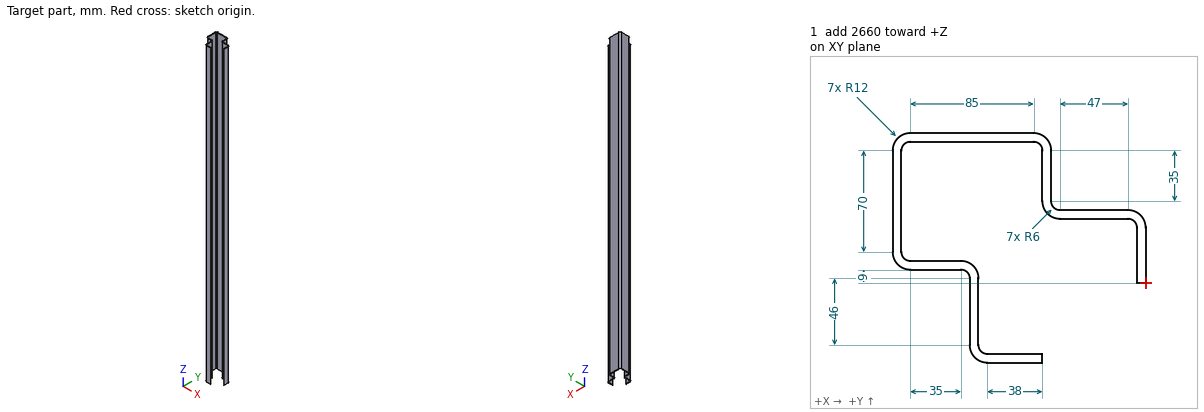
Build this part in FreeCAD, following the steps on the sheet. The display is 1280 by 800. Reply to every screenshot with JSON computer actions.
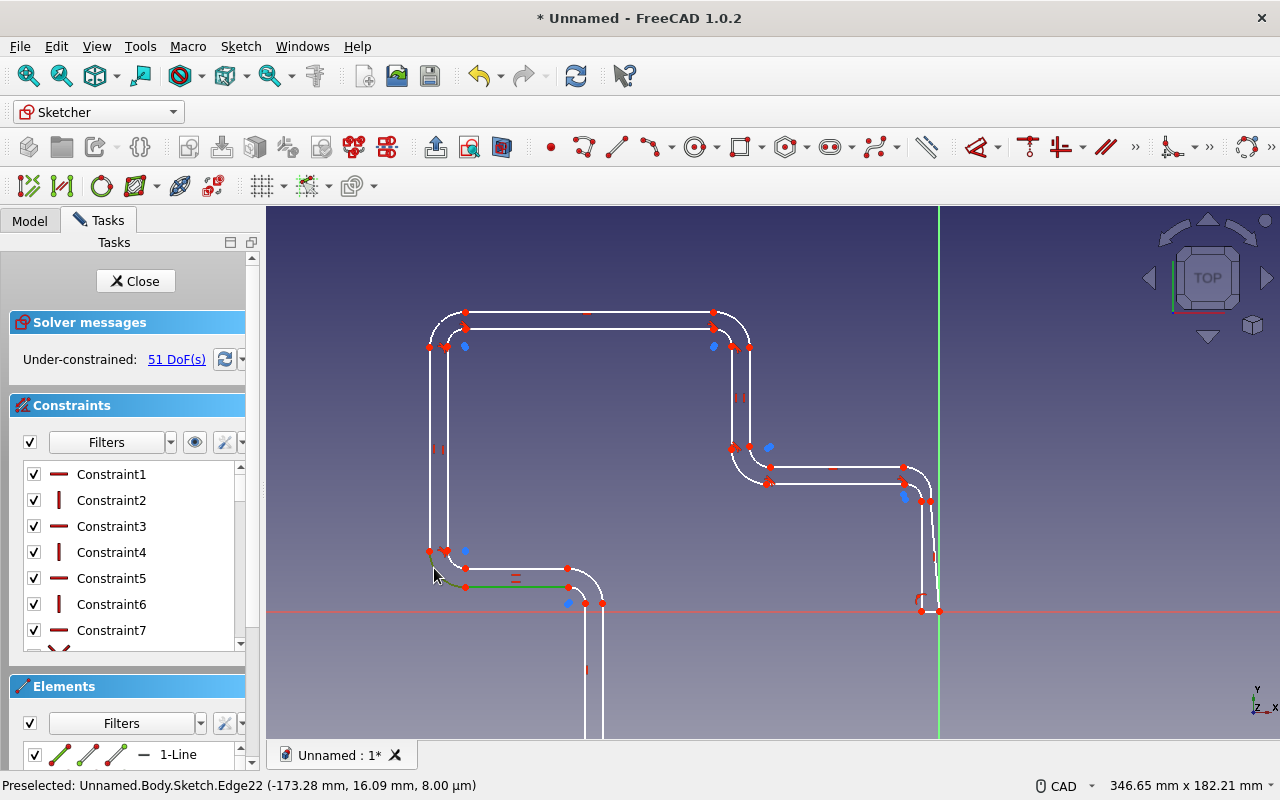
{"action": "key", "text": "t"}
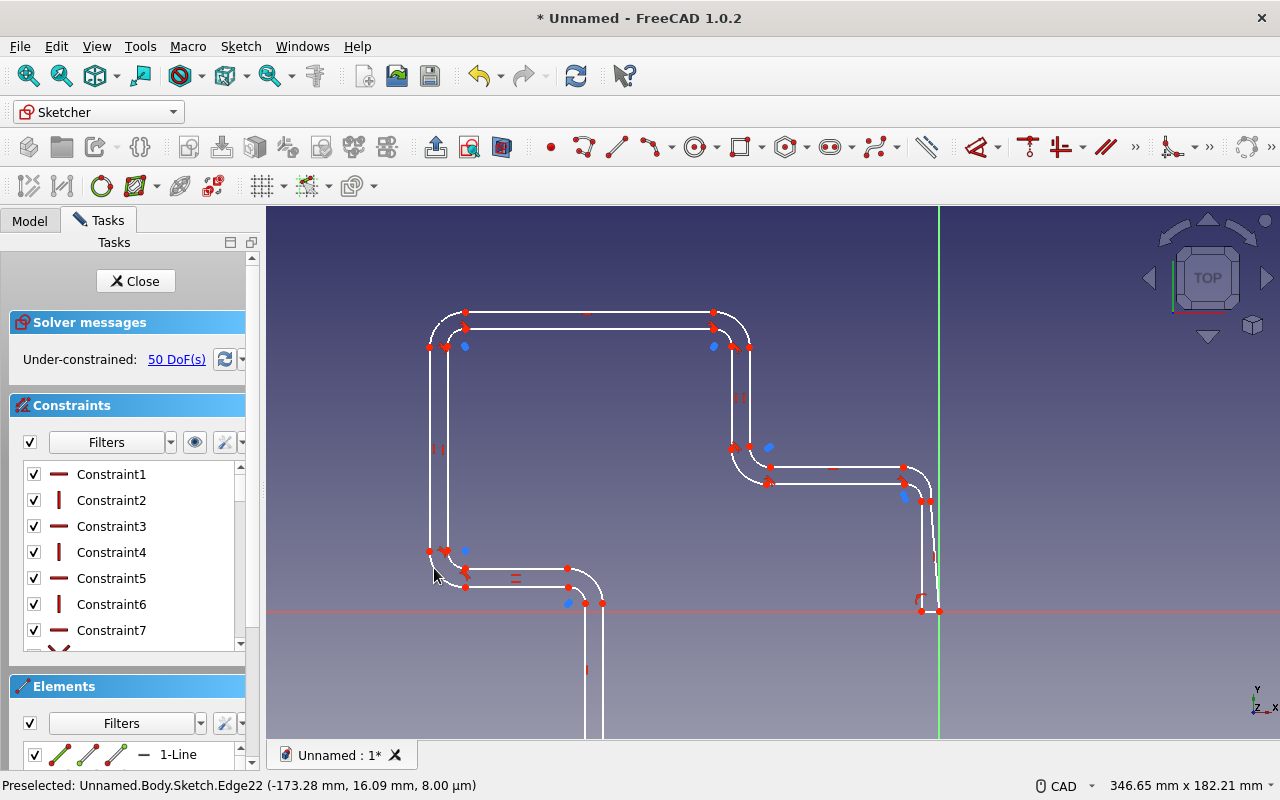
{"action": "left_click", "coordinate": [496, 587]}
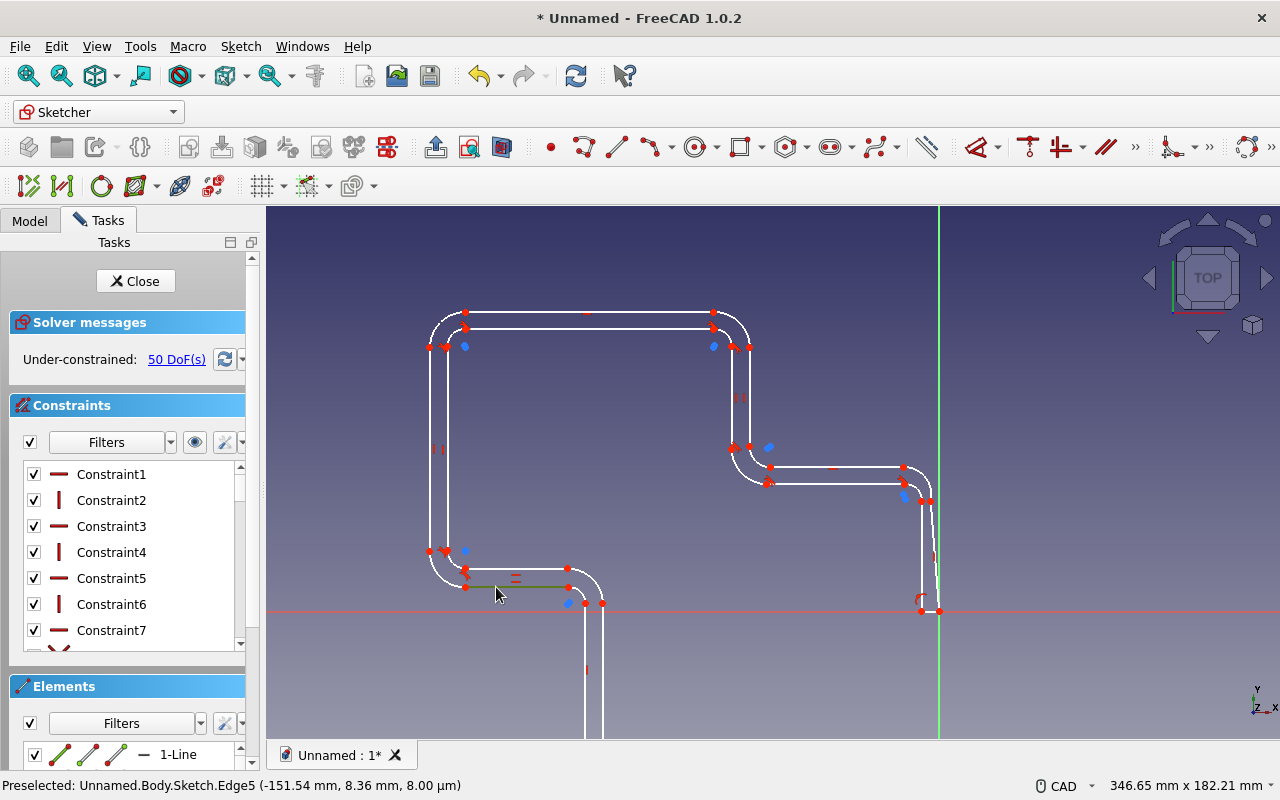
{"action": "left_click", "coordinate": [580, 592]}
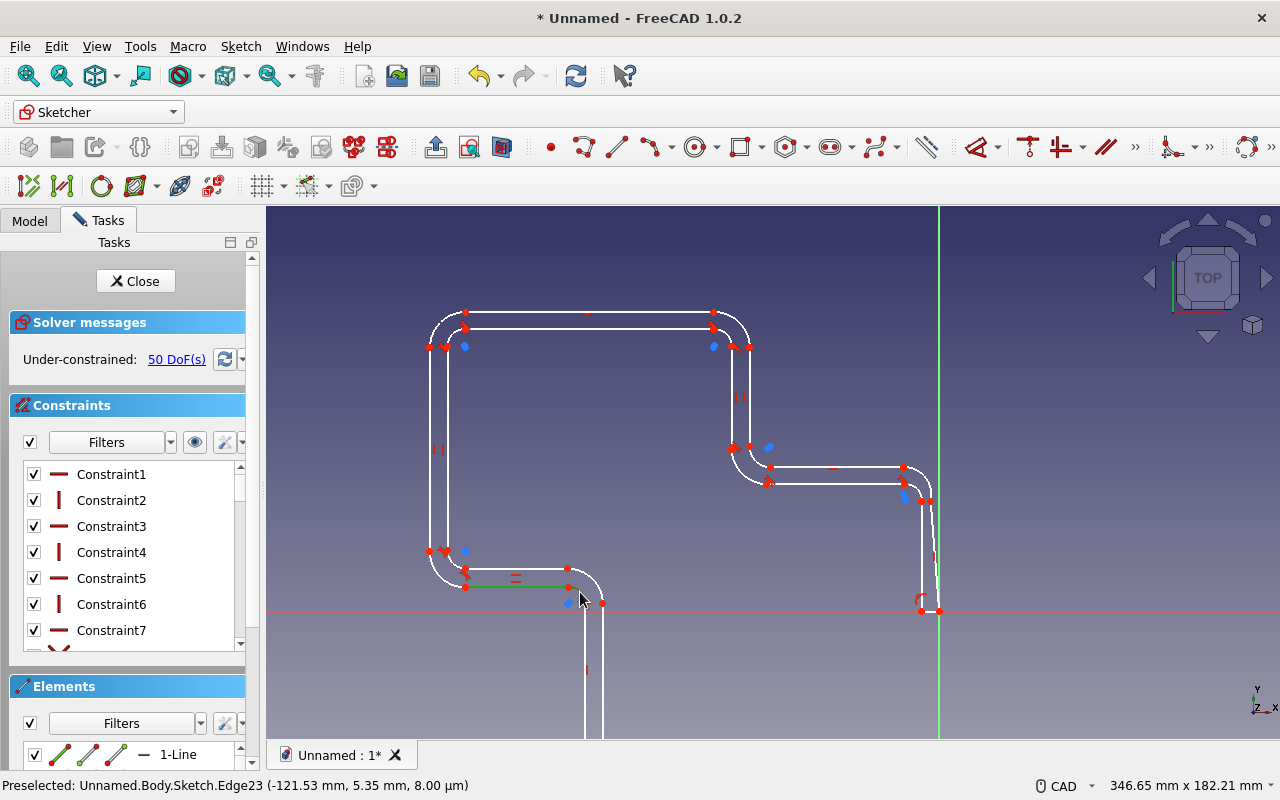
{"action": "key", "text": "t"}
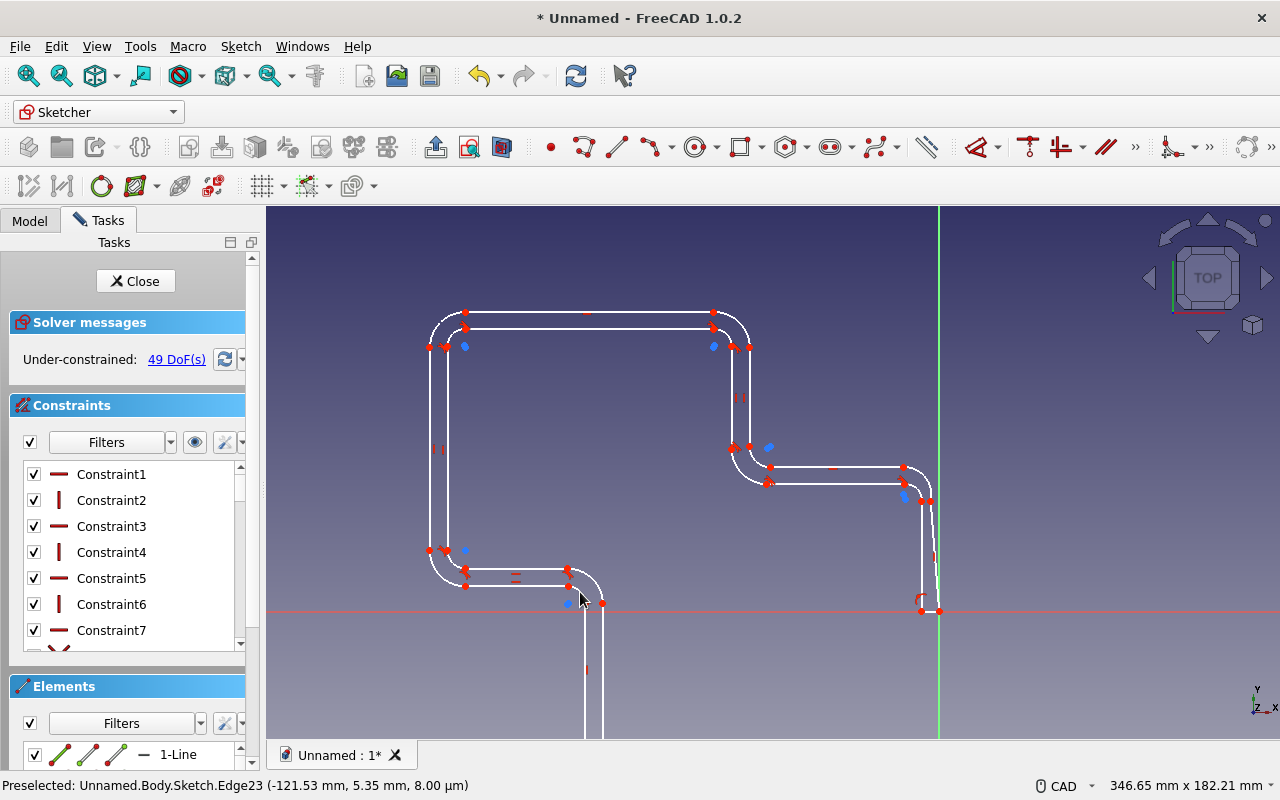
{"action": "left_click", "coordinate": [585, 644]}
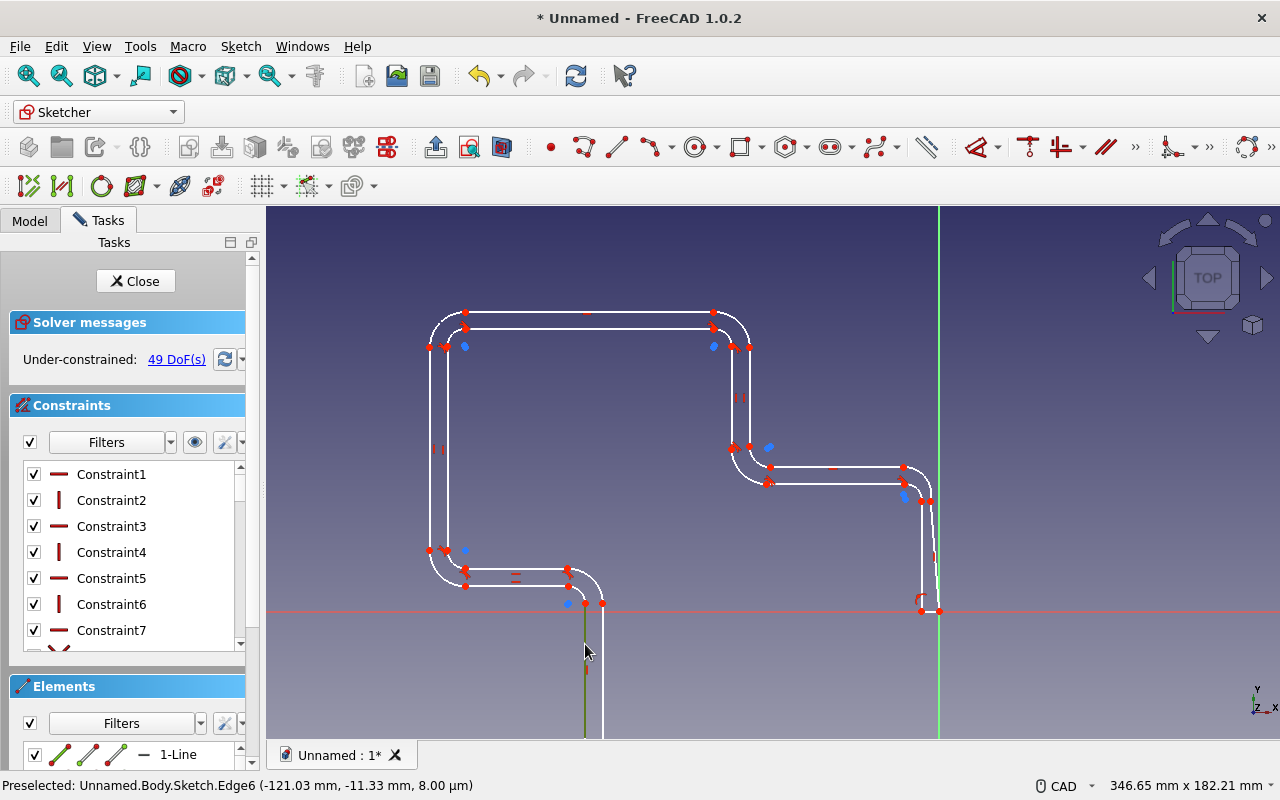
{"action": "left_click", "coordinate": [580, 591]}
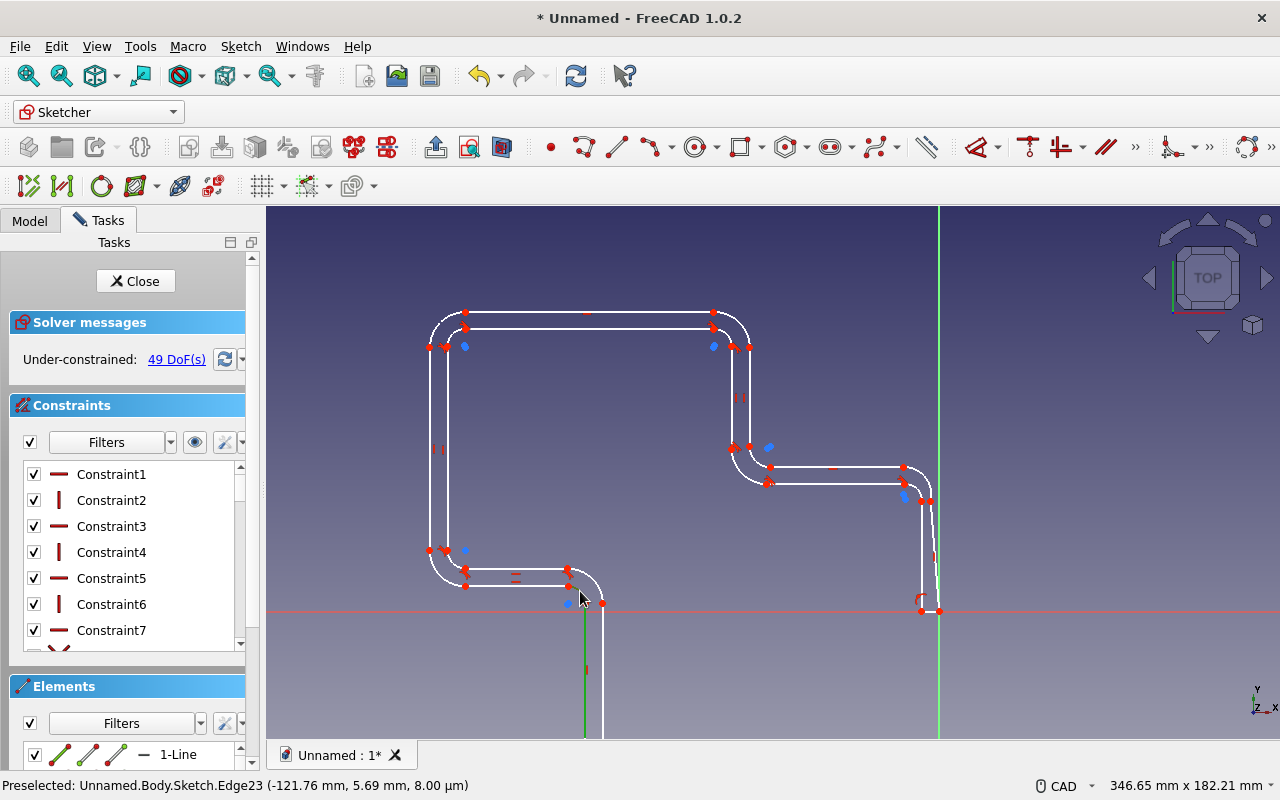
{"action": "key", "text": "t"}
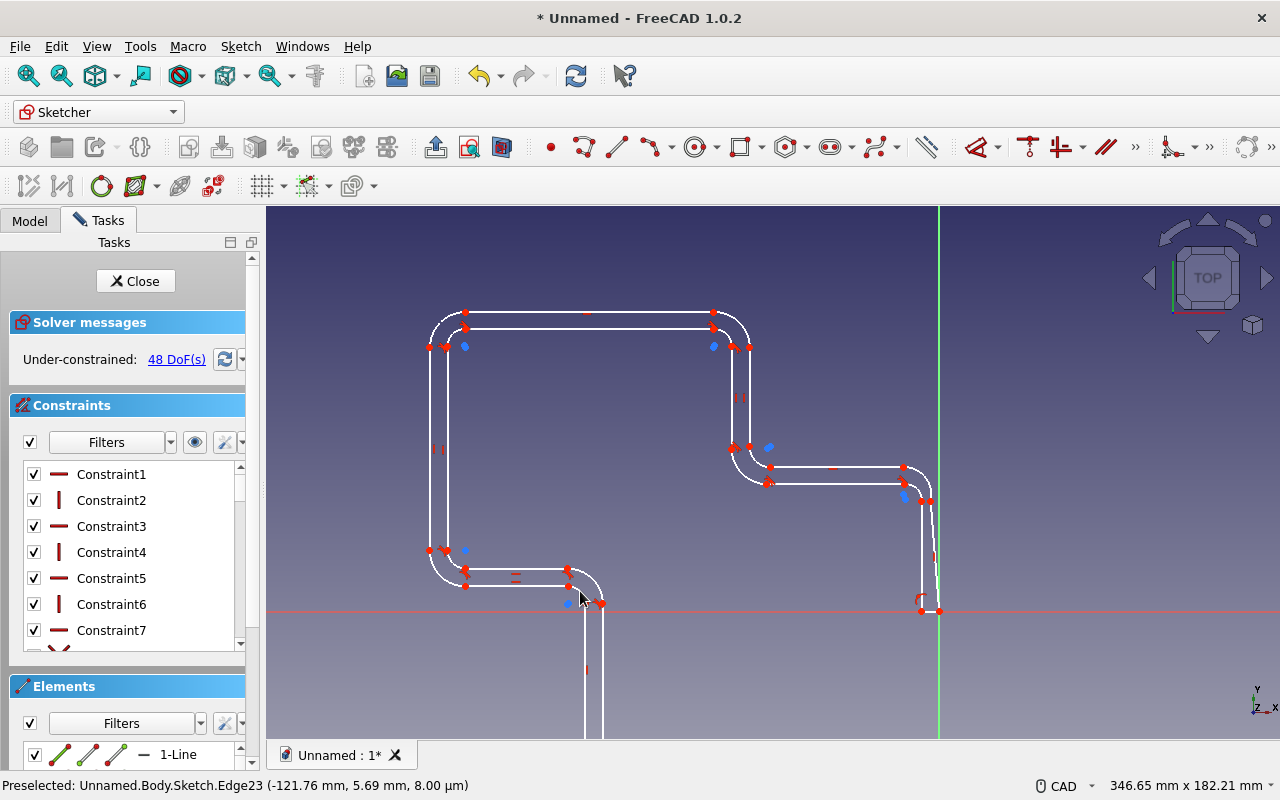
{"action": "left_click", "coordinate": [585, 644]}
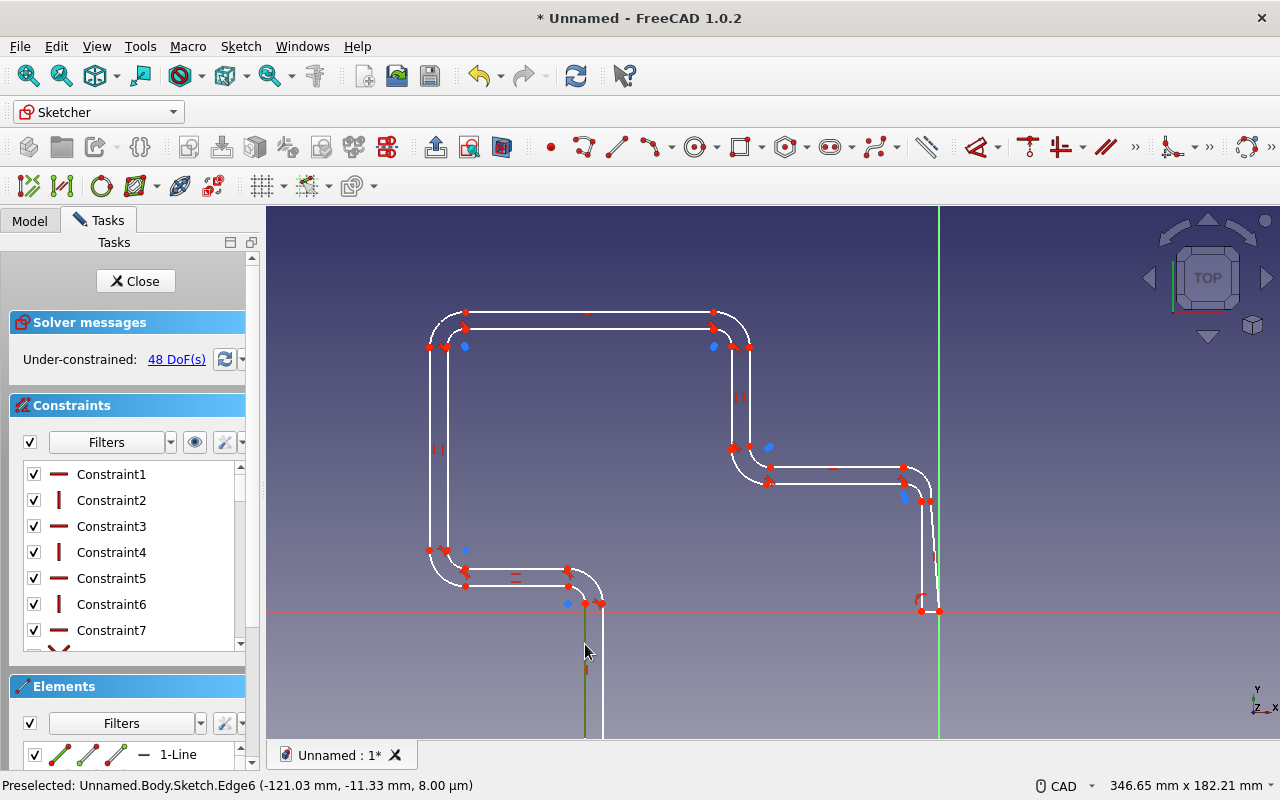
{"action": "scroll", "coordinate": [745, 332], "scroll_direction": "down", "scroll_amount": 2}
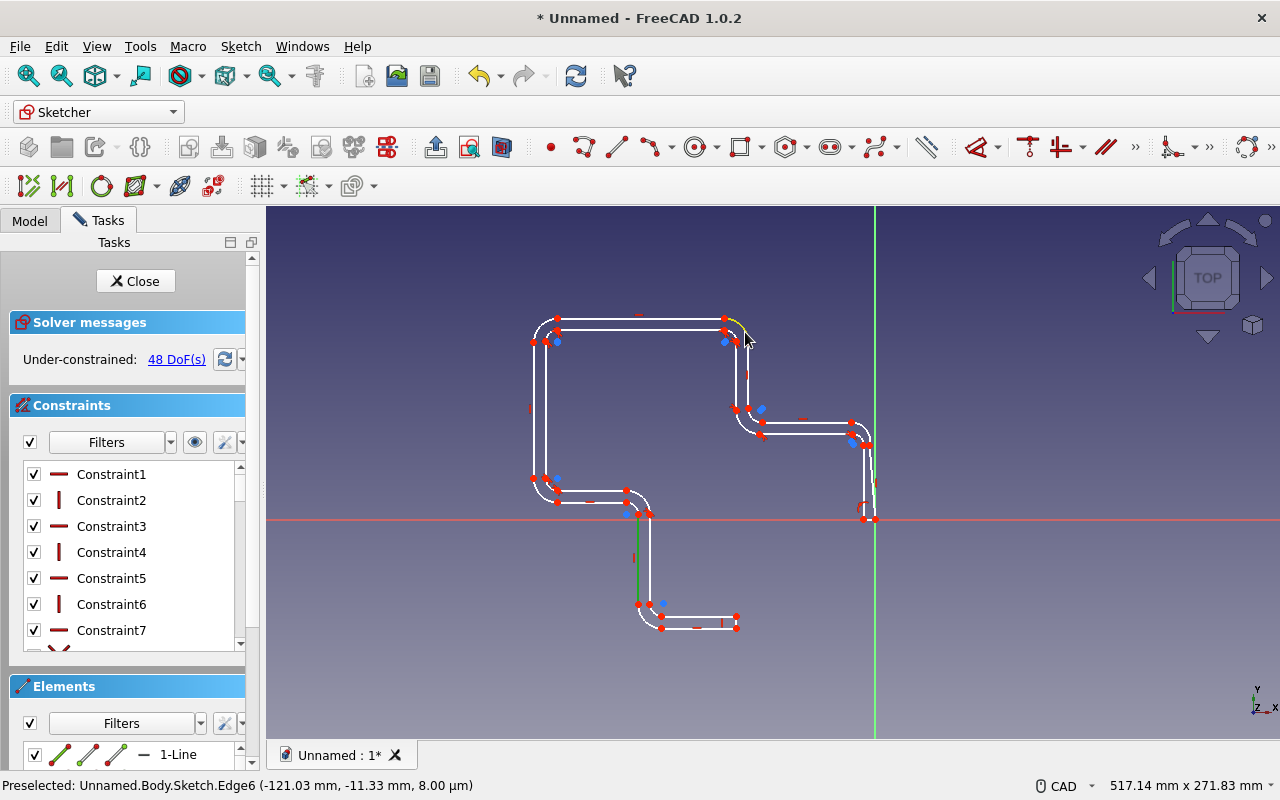
{"action": "scroll", "coordinate": [641, 615], "scroll_direction": "up", "scroll_amount": 2}